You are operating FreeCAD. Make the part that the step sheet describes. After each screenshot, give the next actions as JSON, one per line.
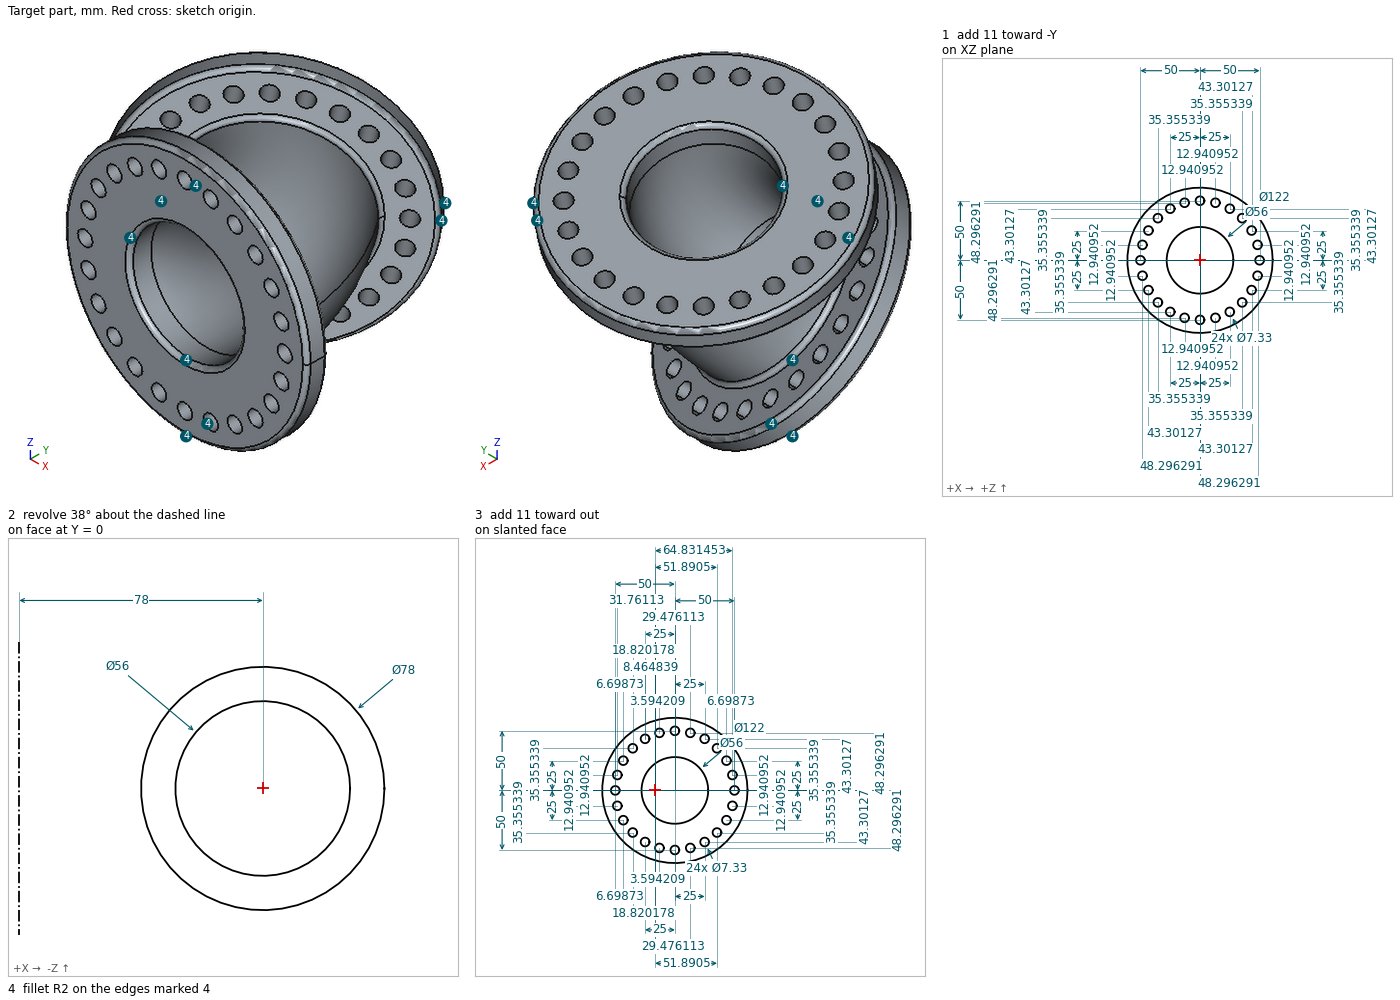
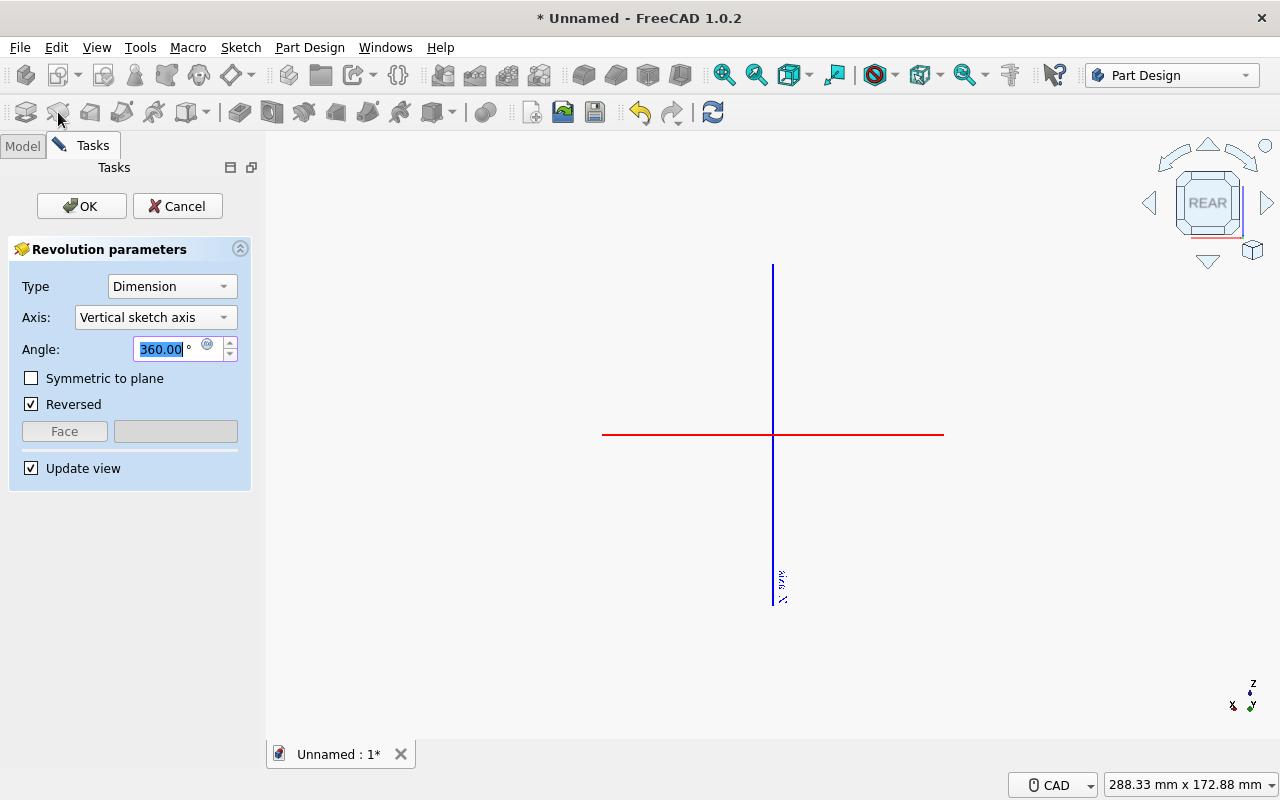
{"action": "left_click", "coordinate": [156, 318]}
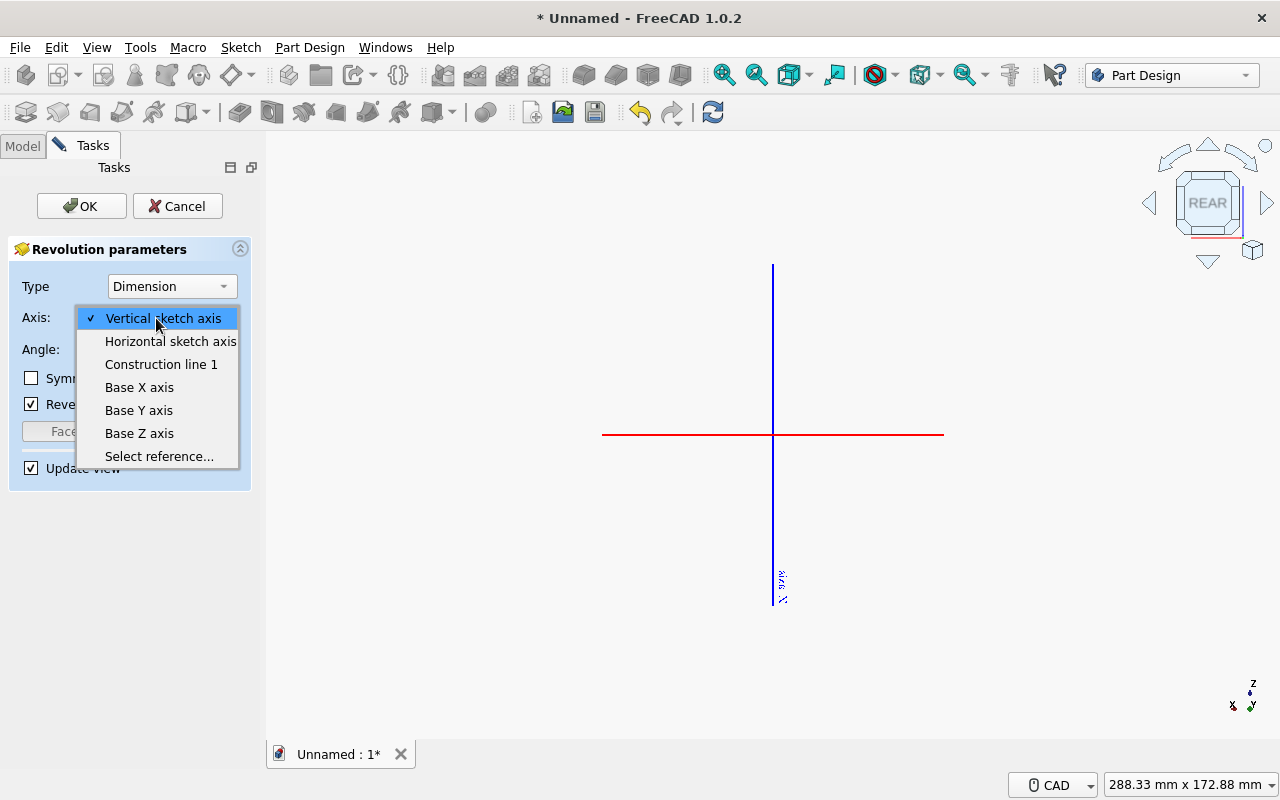
{"action": "left_click", "coordinate": [156, 364]}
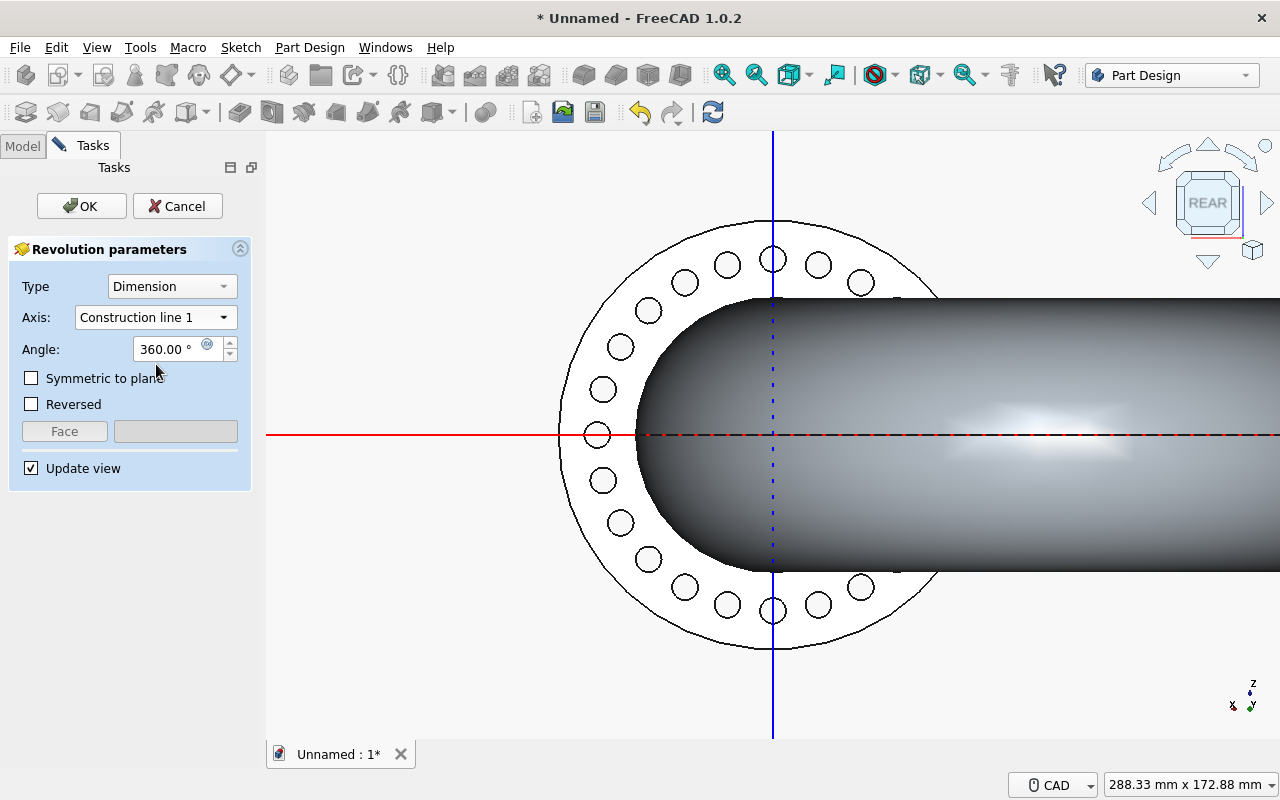
{"action": "triple_click", "coordinate": [178, 349]}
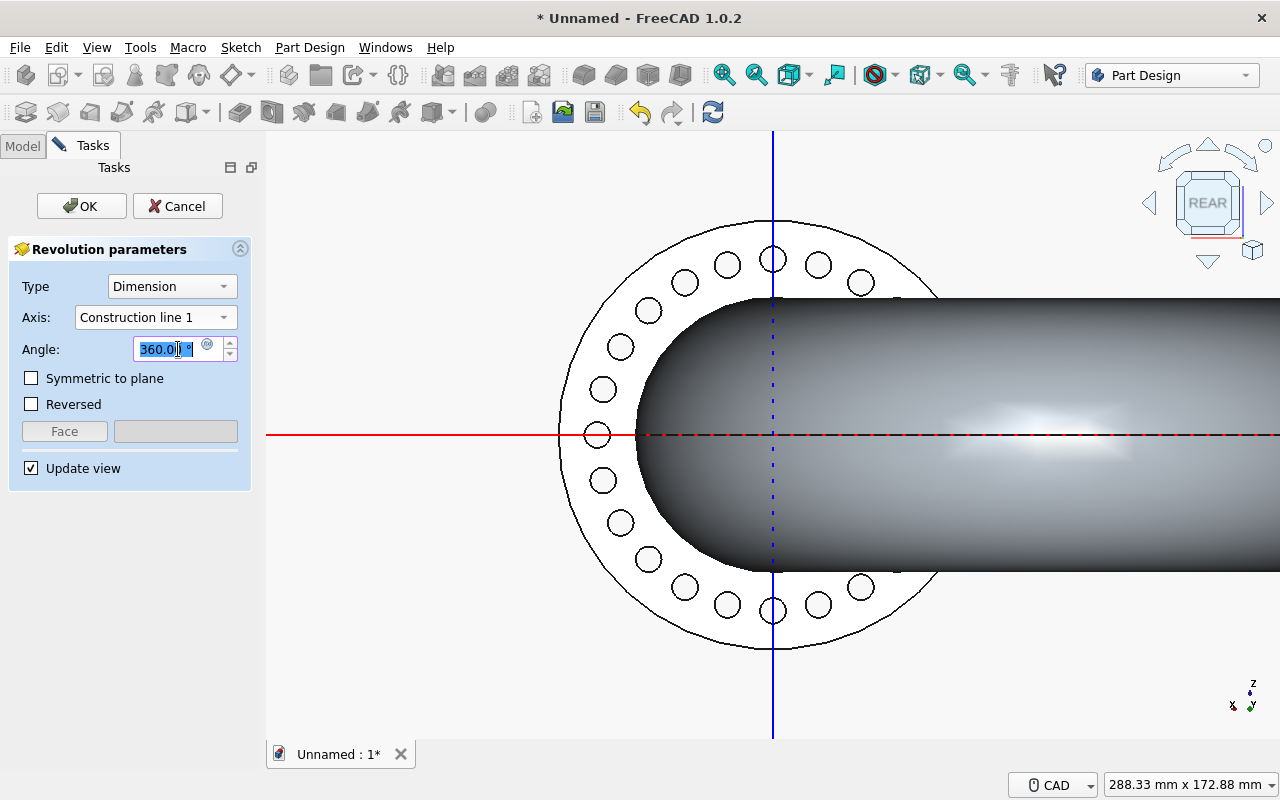
{"action": "type", "text": "38"}
{"action": "key", "text": "Tab"}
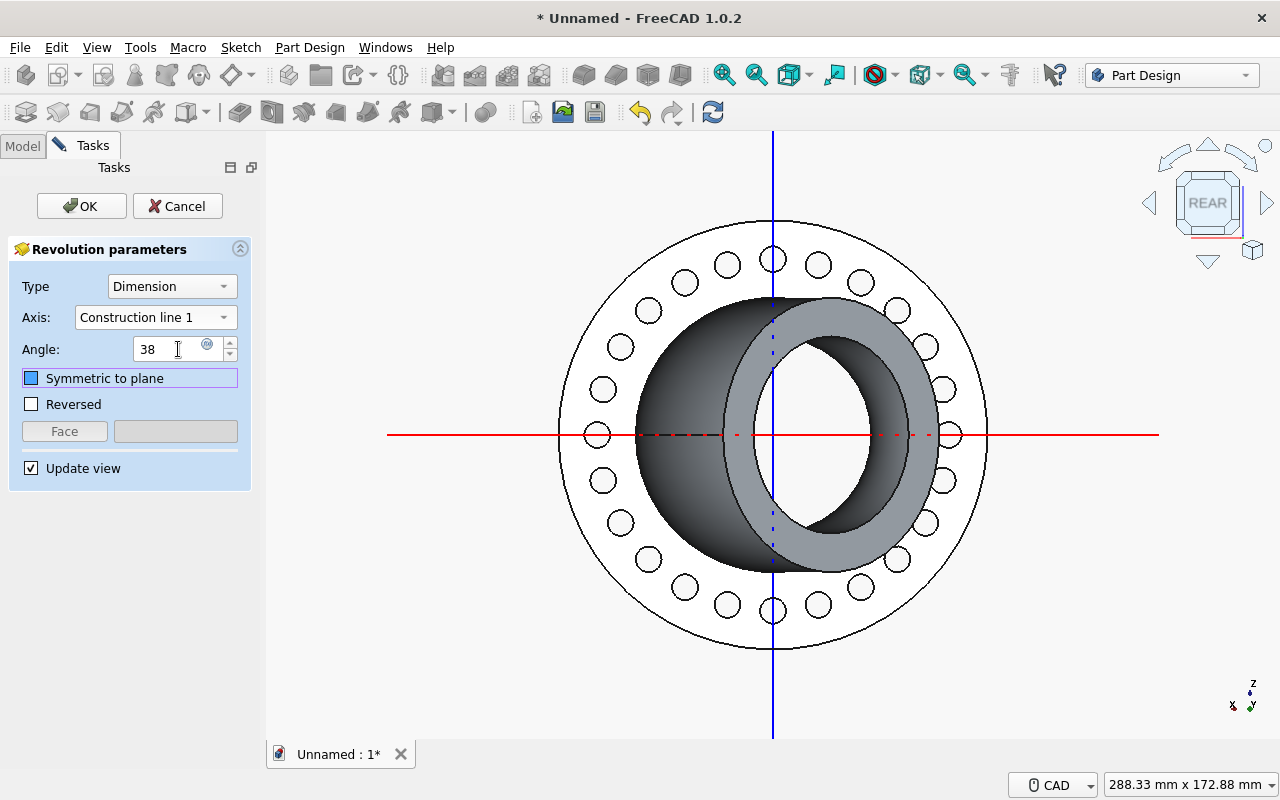
{"action": "left_click", "coordinate": [82, 206]}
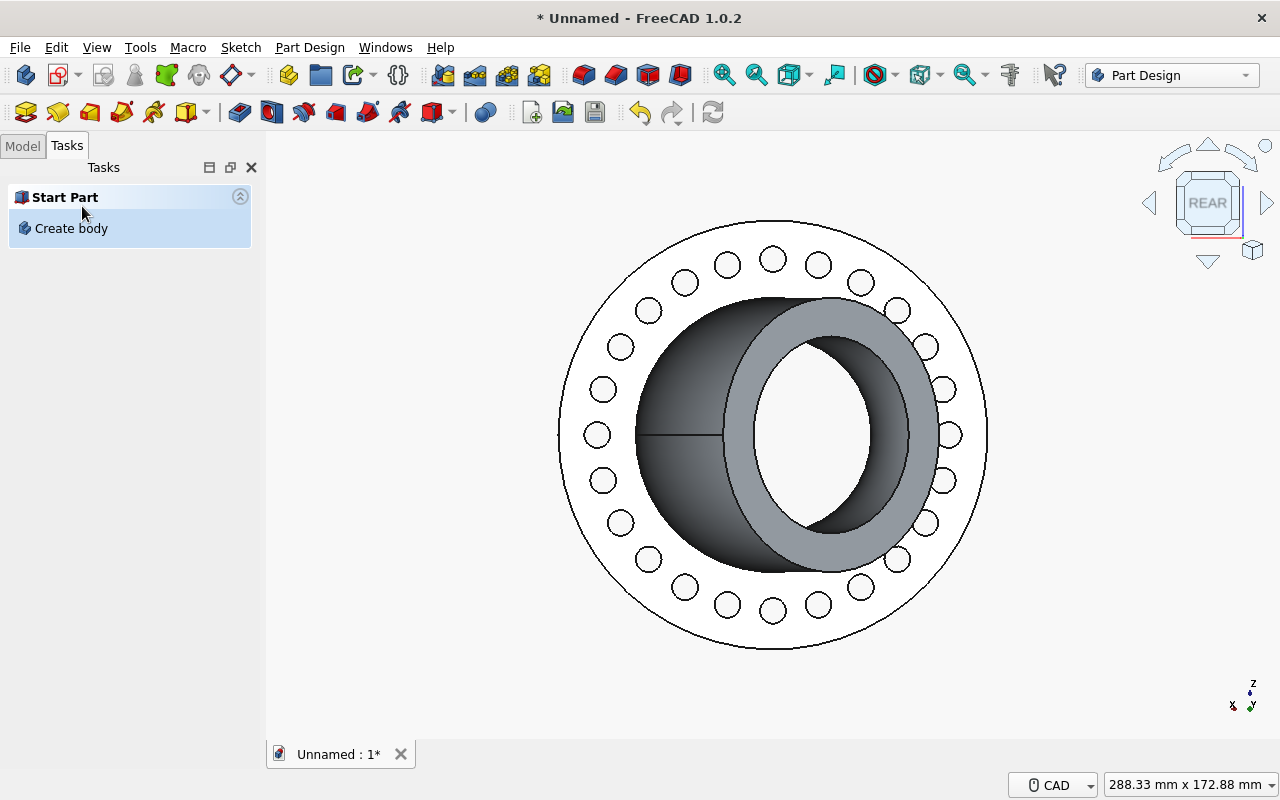
{"action": "left_click", "coordinate": [831, 316]}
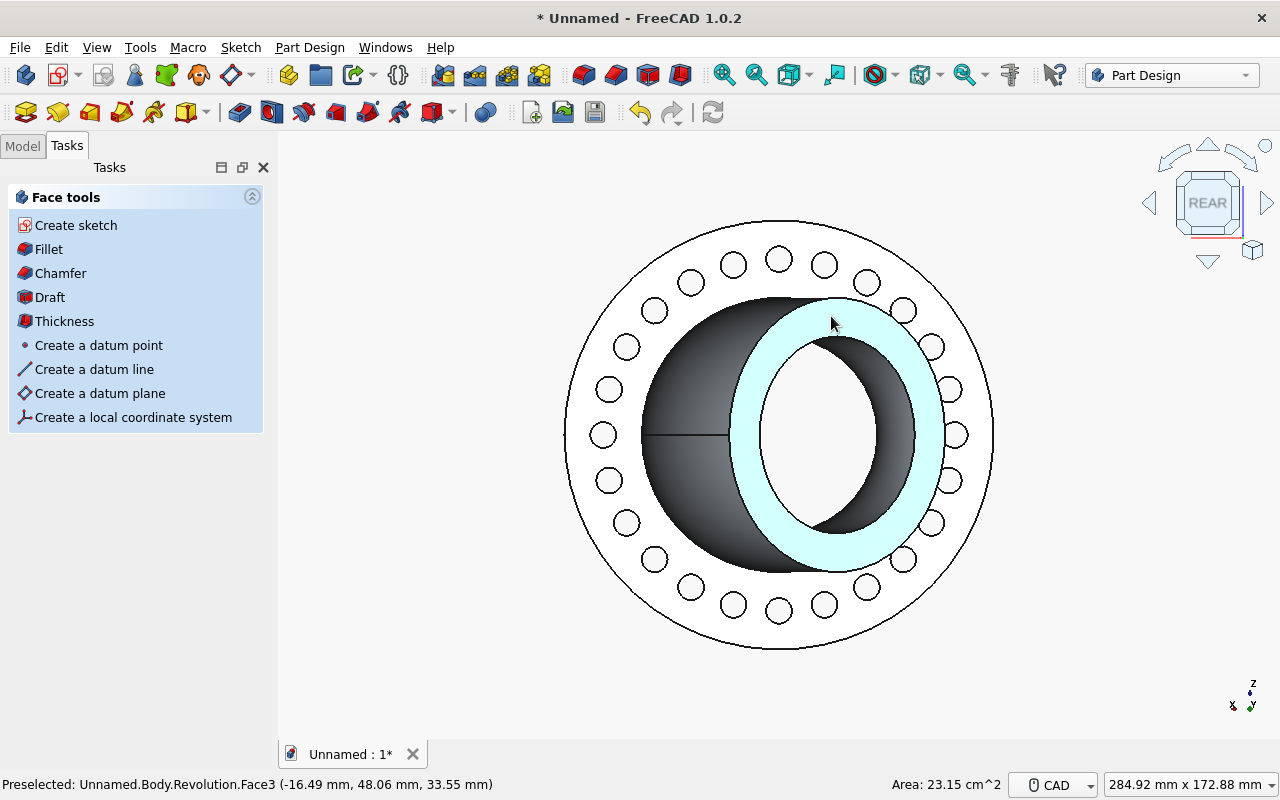
{"action": "left_click", "coordinate": [58, 76]}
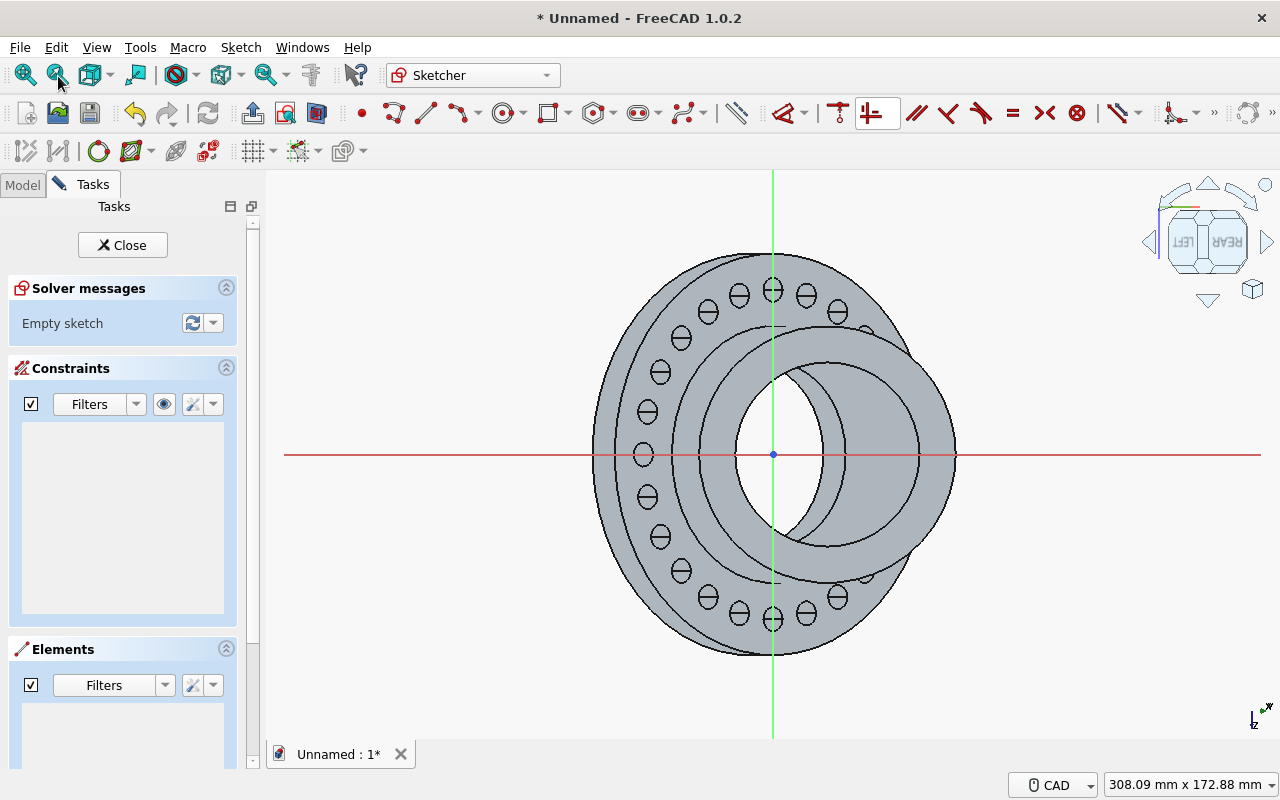
{"action": "left_click", "coordinate": [504, 114]}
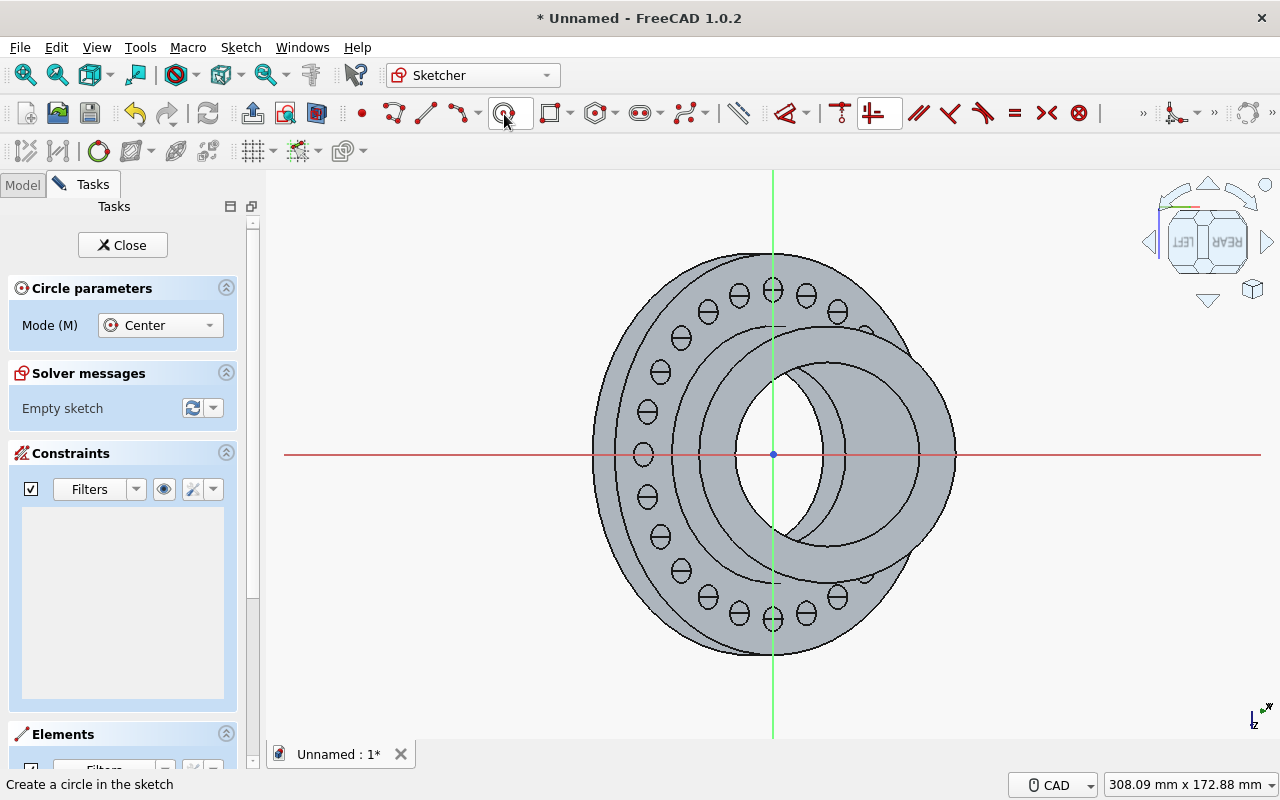
{"action": "left_click", "coordinate": [827, 454]}
{"action": "left_click", "coordinate": [969, 313]}